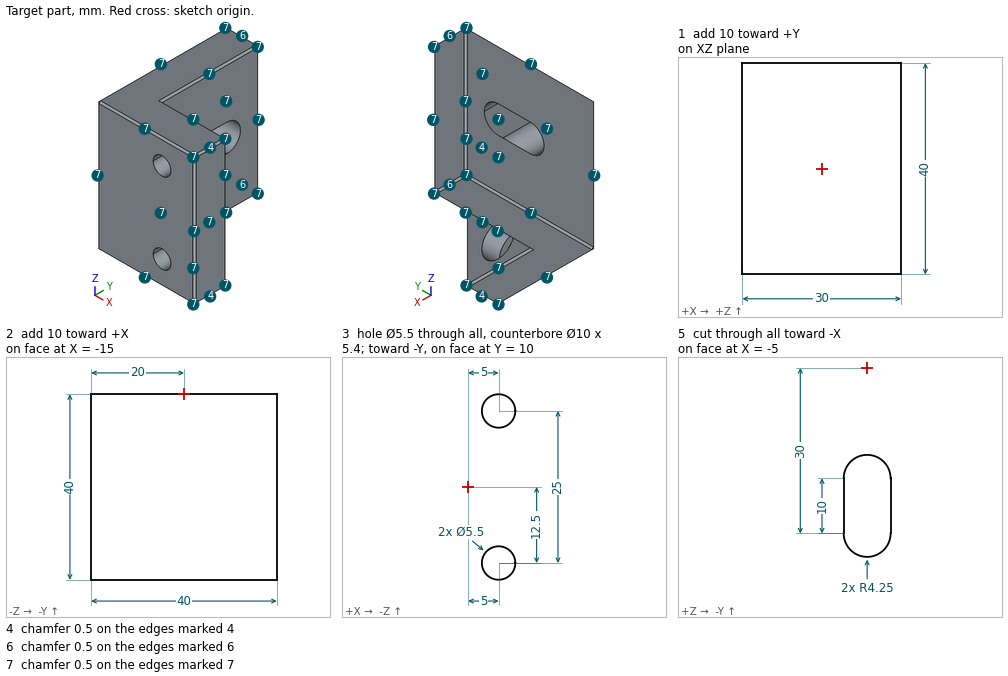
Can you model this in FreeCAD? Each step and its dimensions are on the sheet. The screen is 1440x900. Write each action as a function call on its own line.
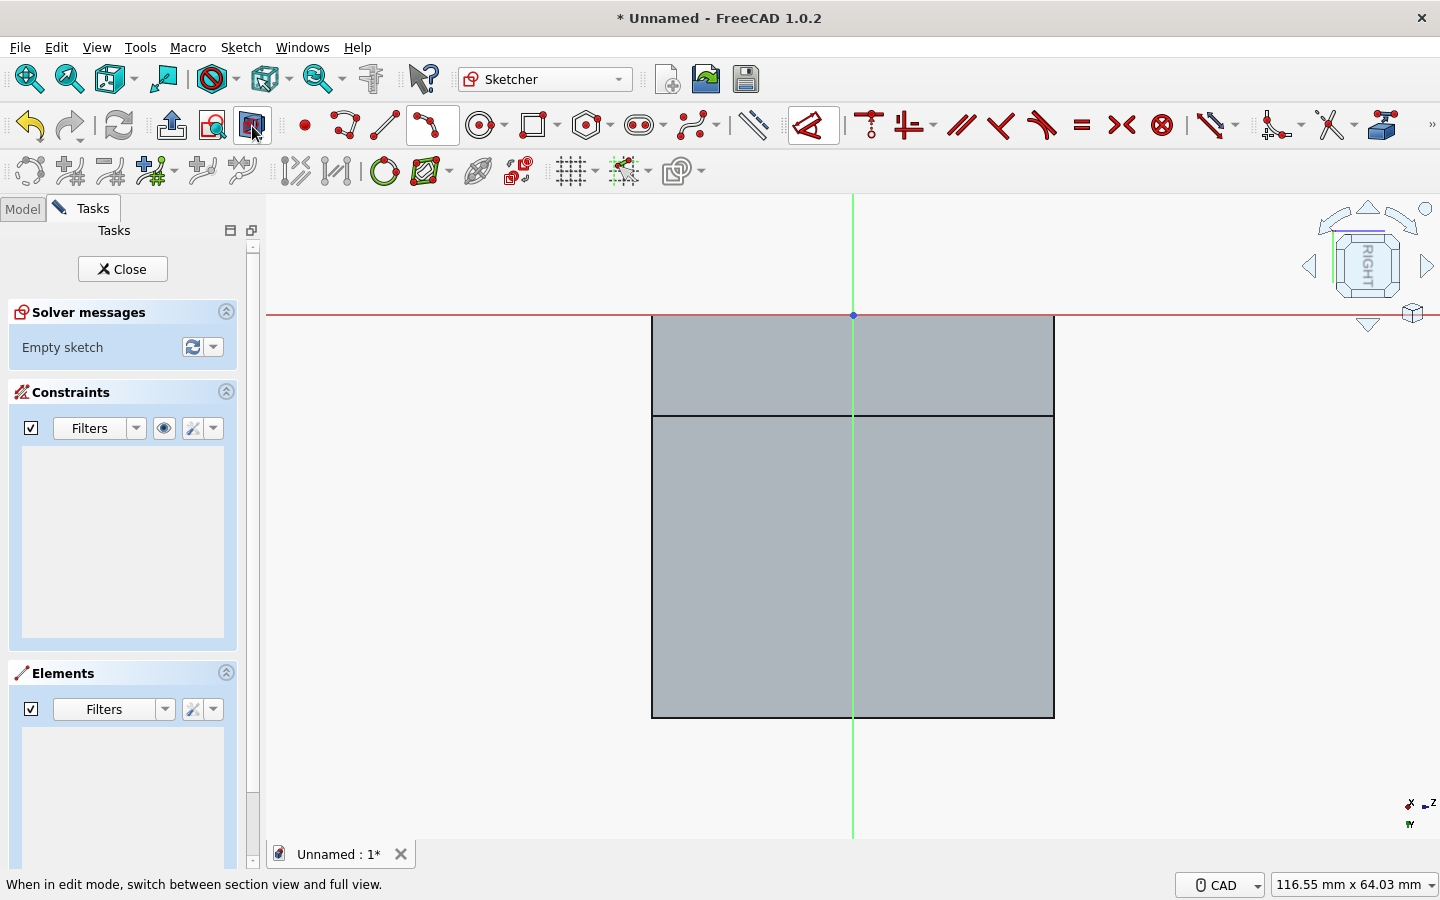
click(640, 126)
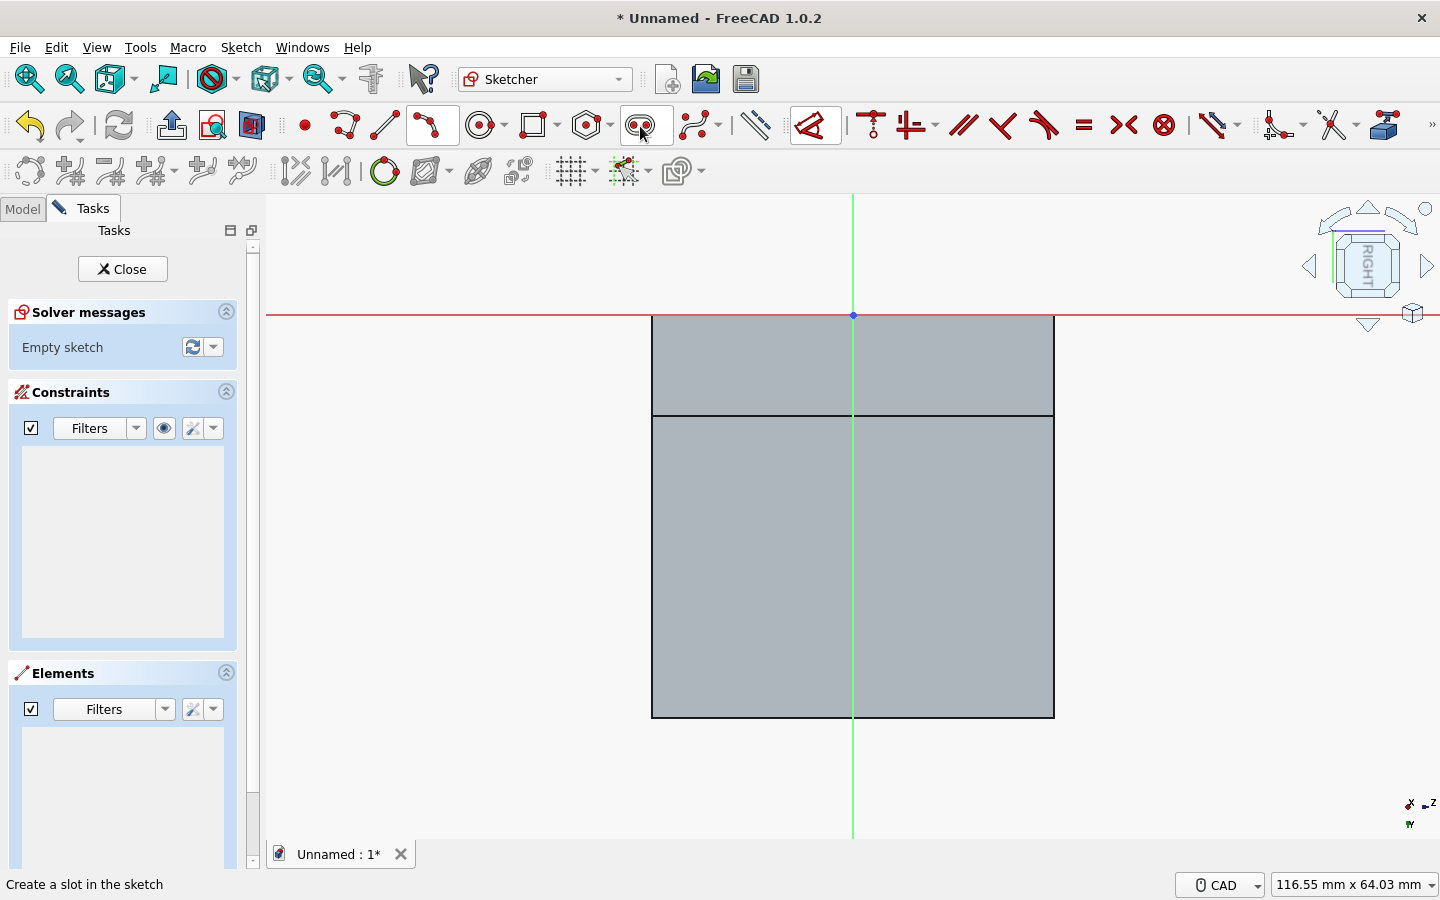
click(853, 617)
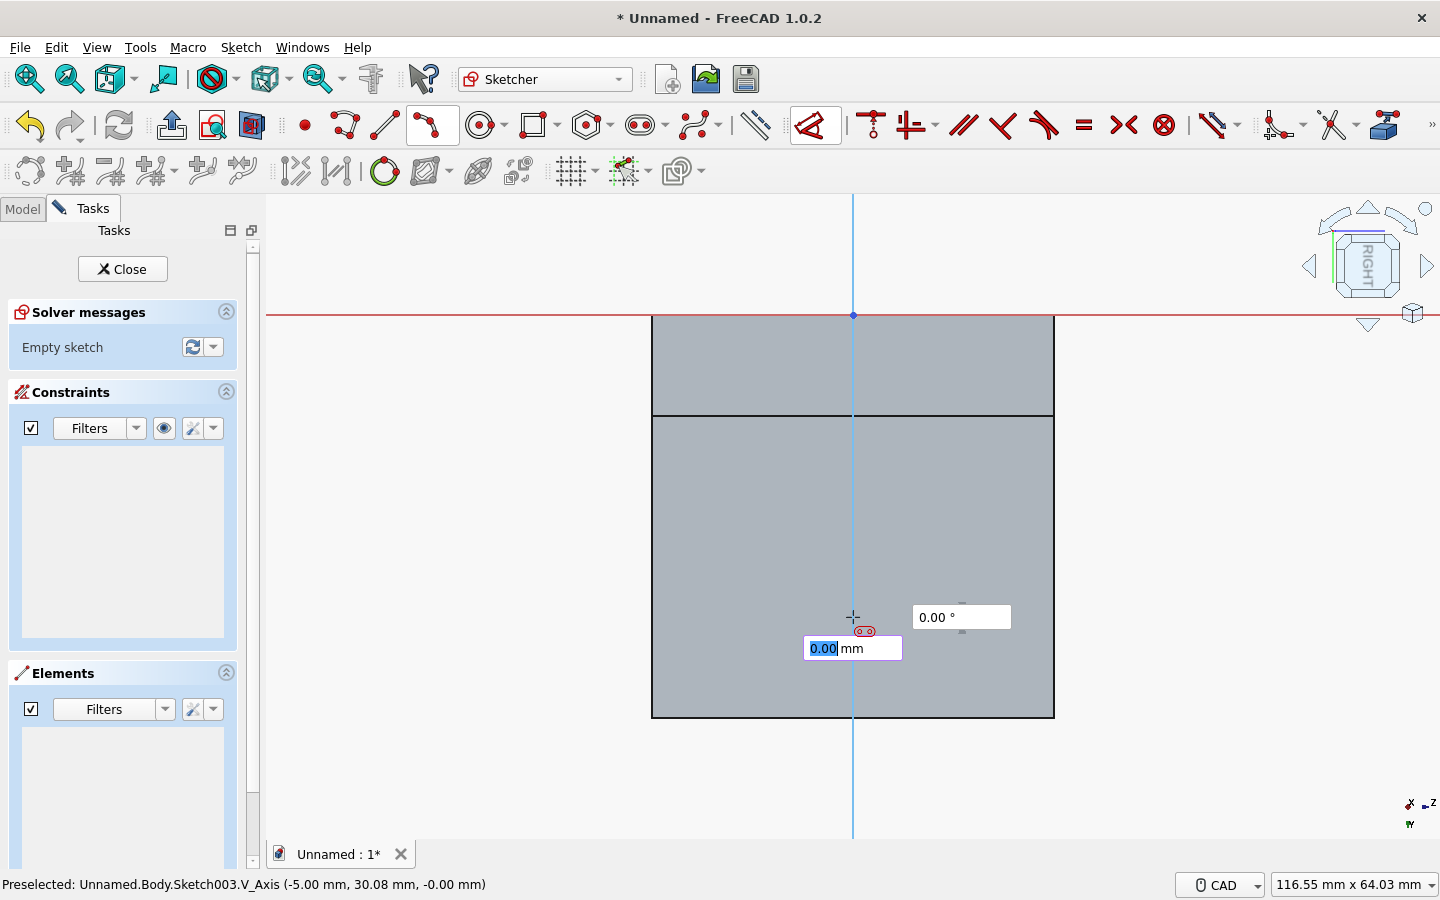
click(862, 517)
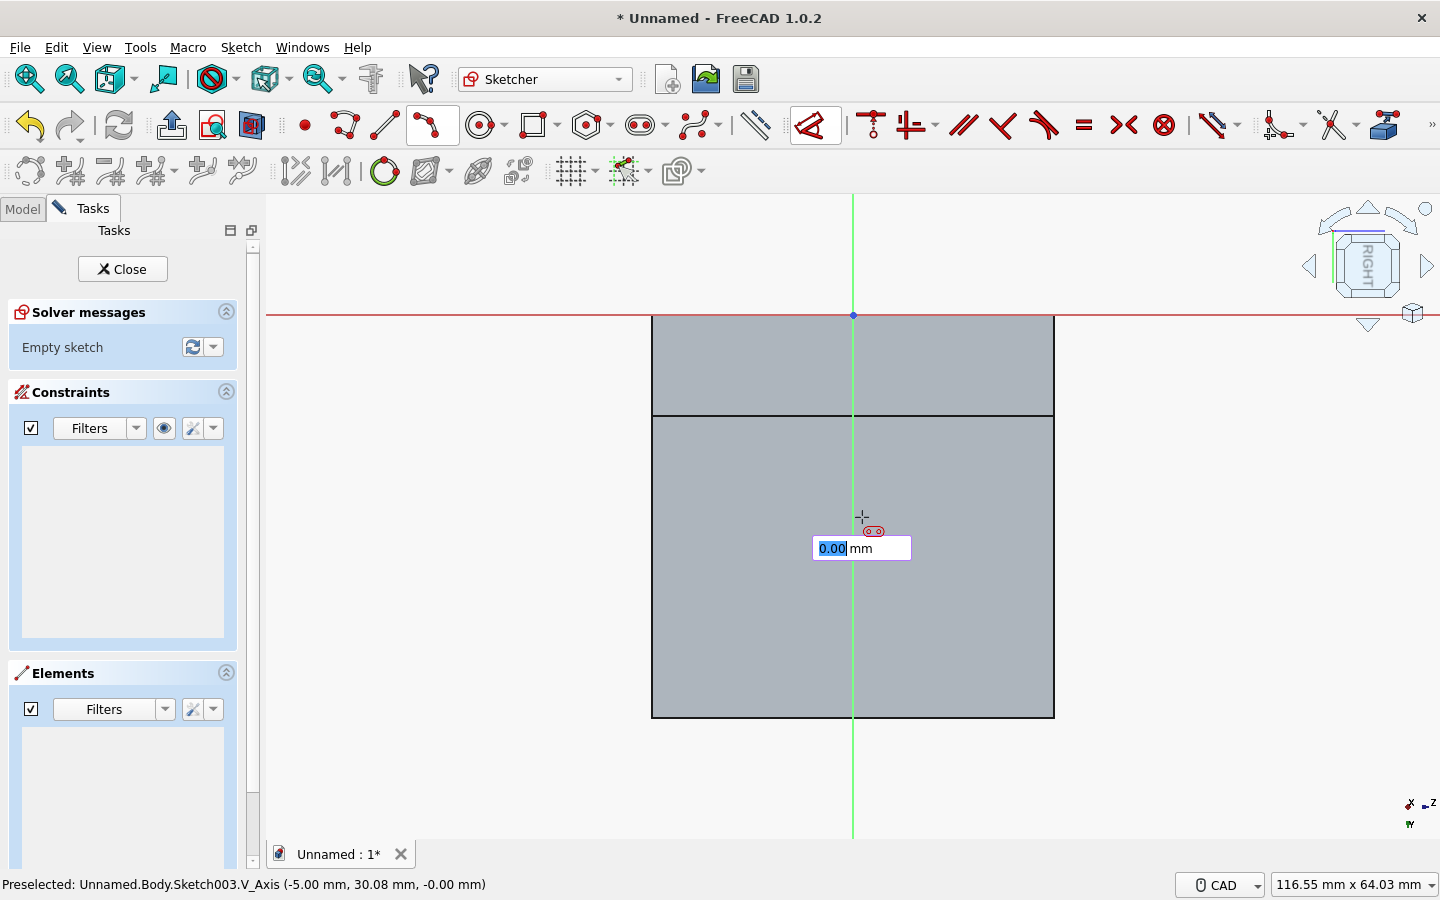
click(810, 567)
key(Escape)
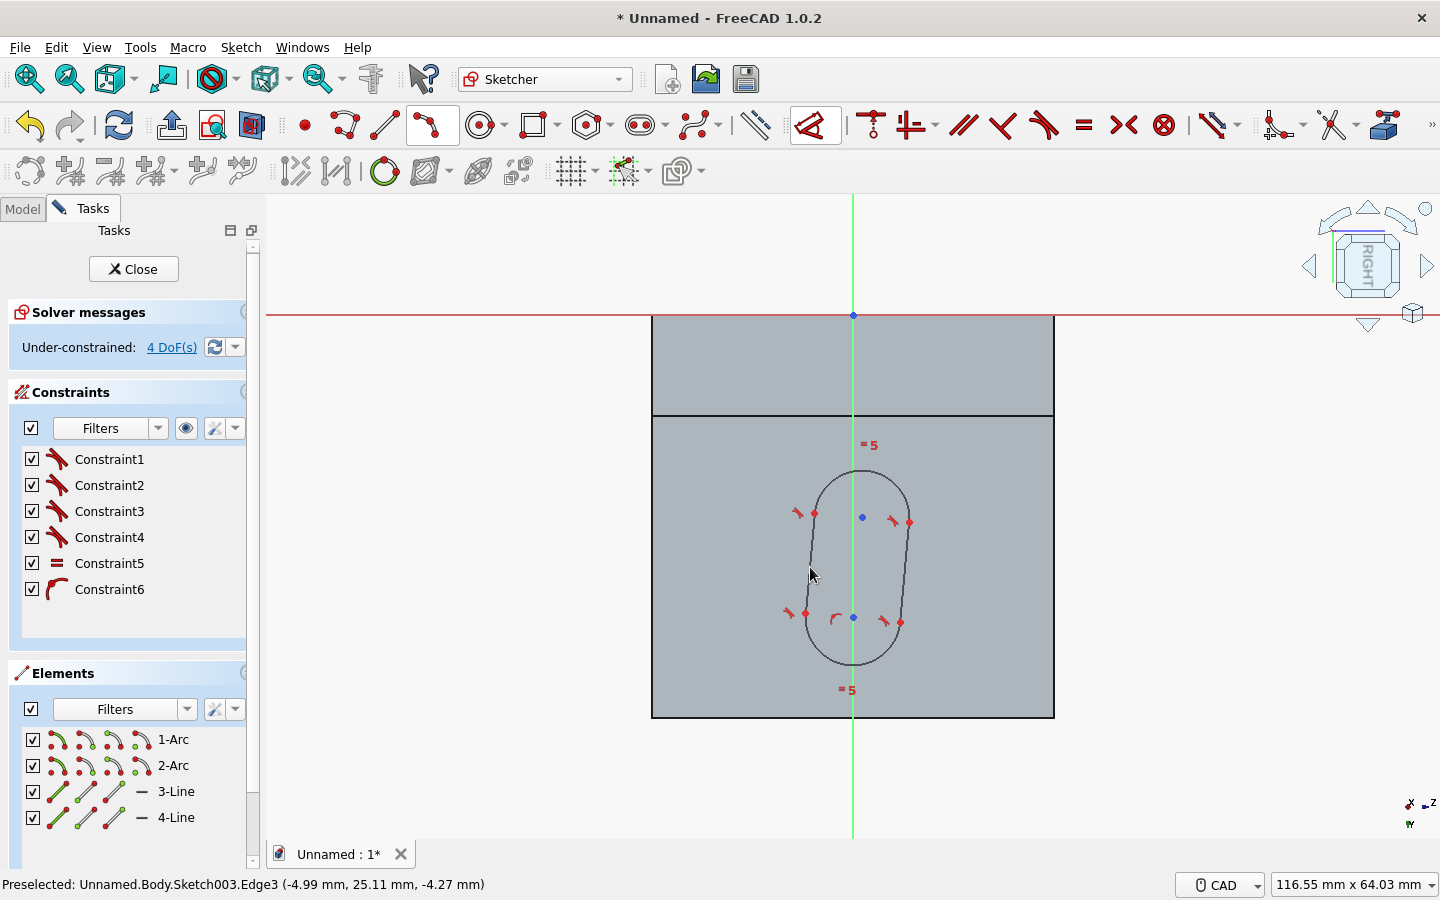
click(809, 584)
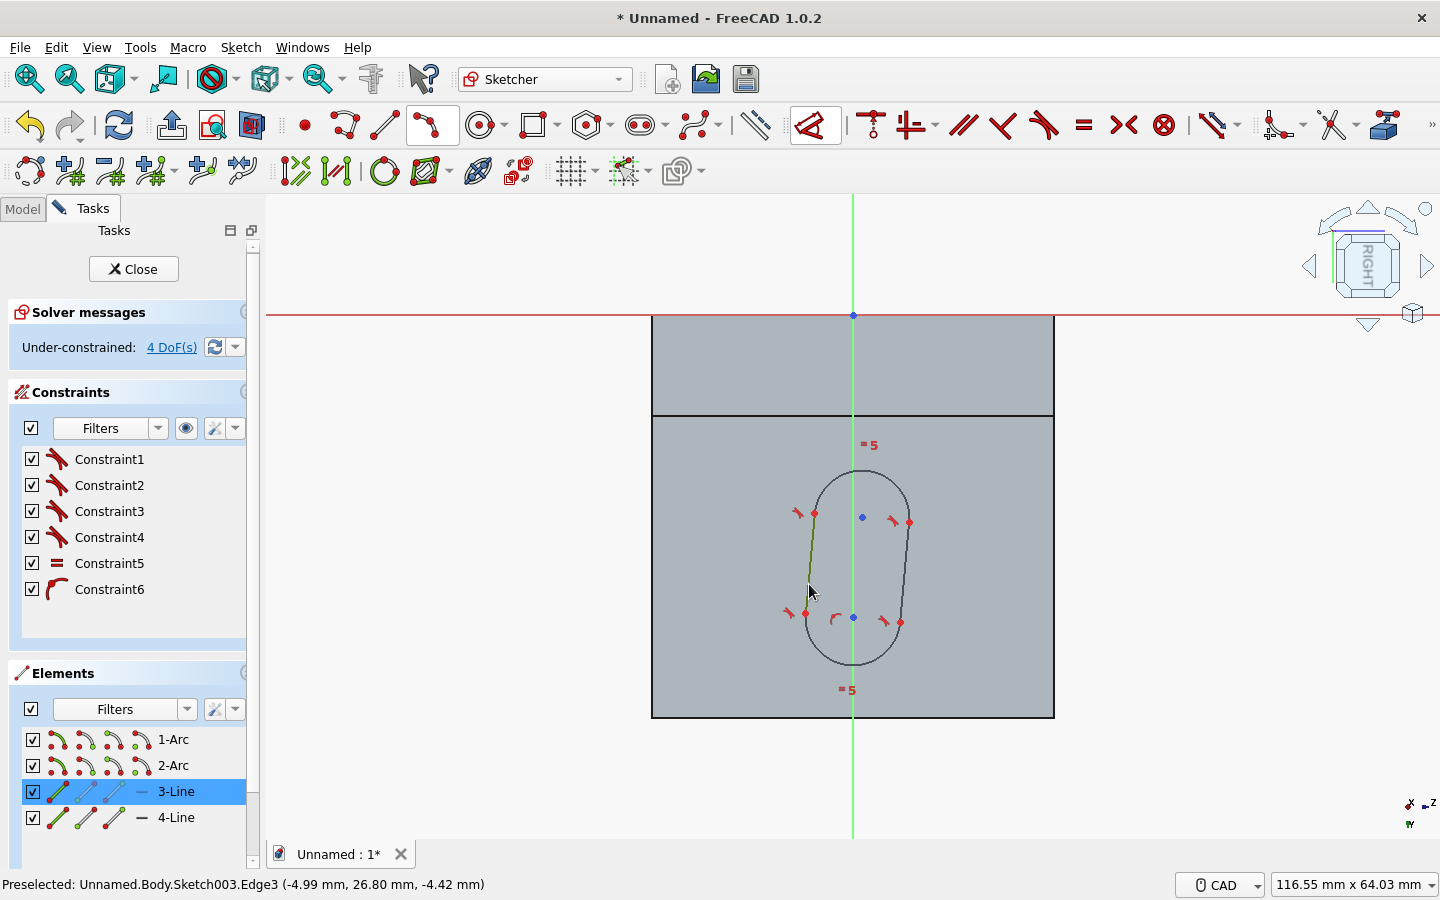
click(938, 126)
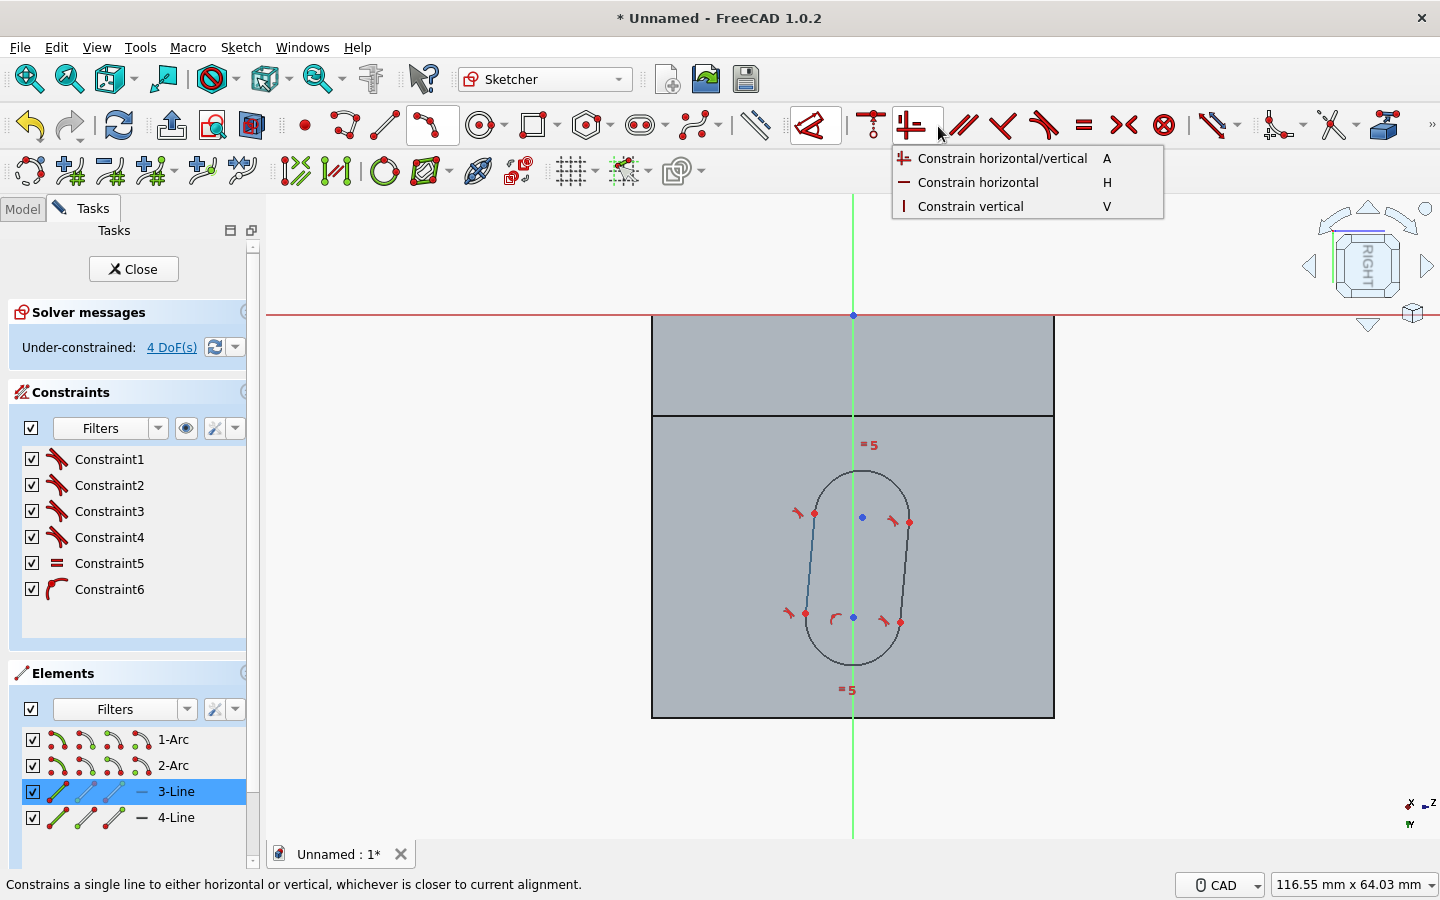
click(1028, 206)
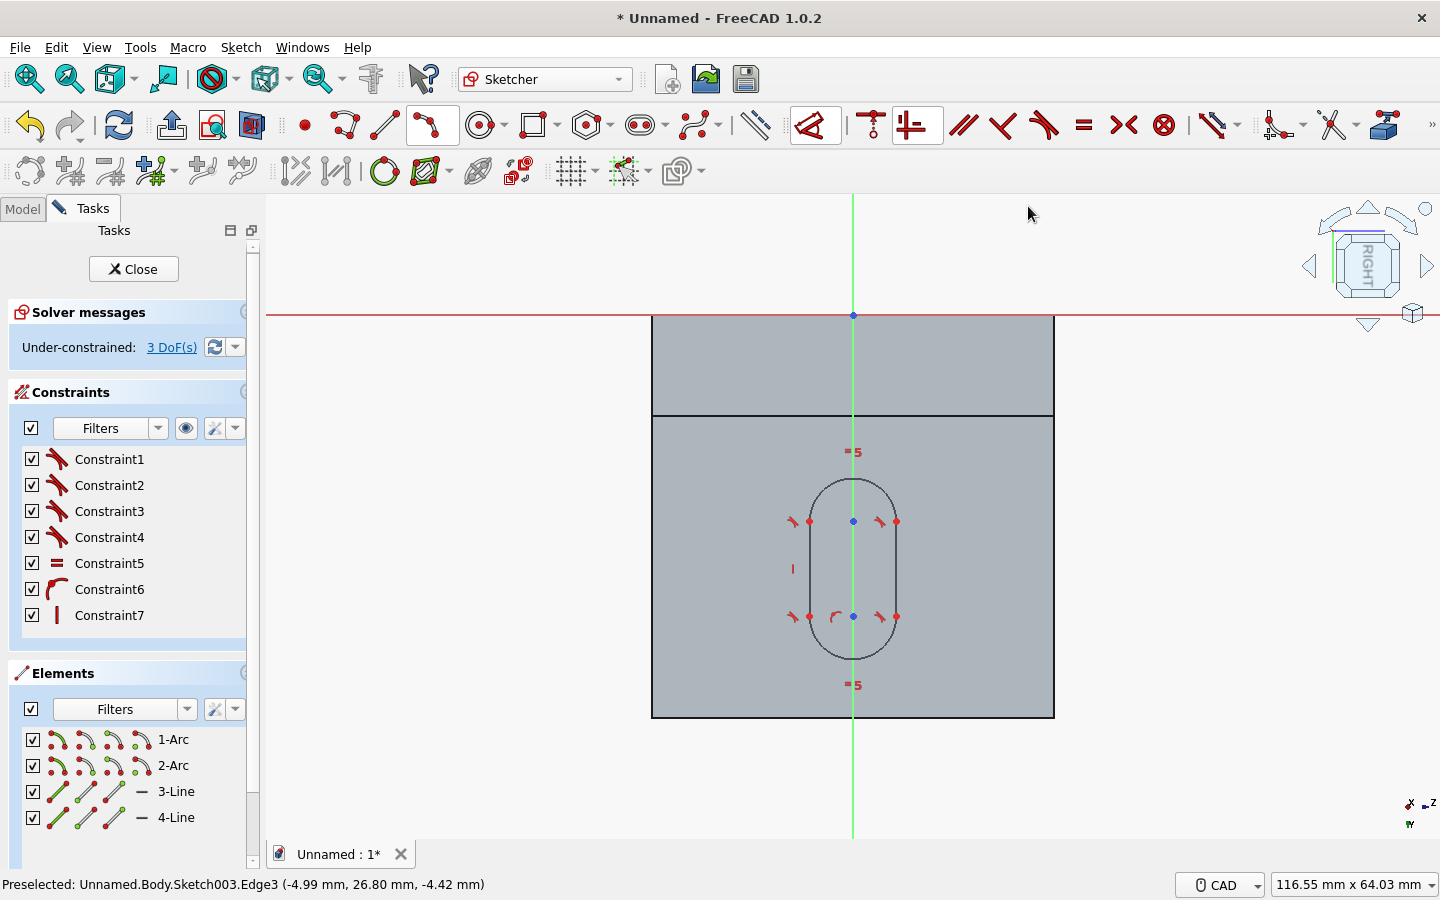
click(828, 651)